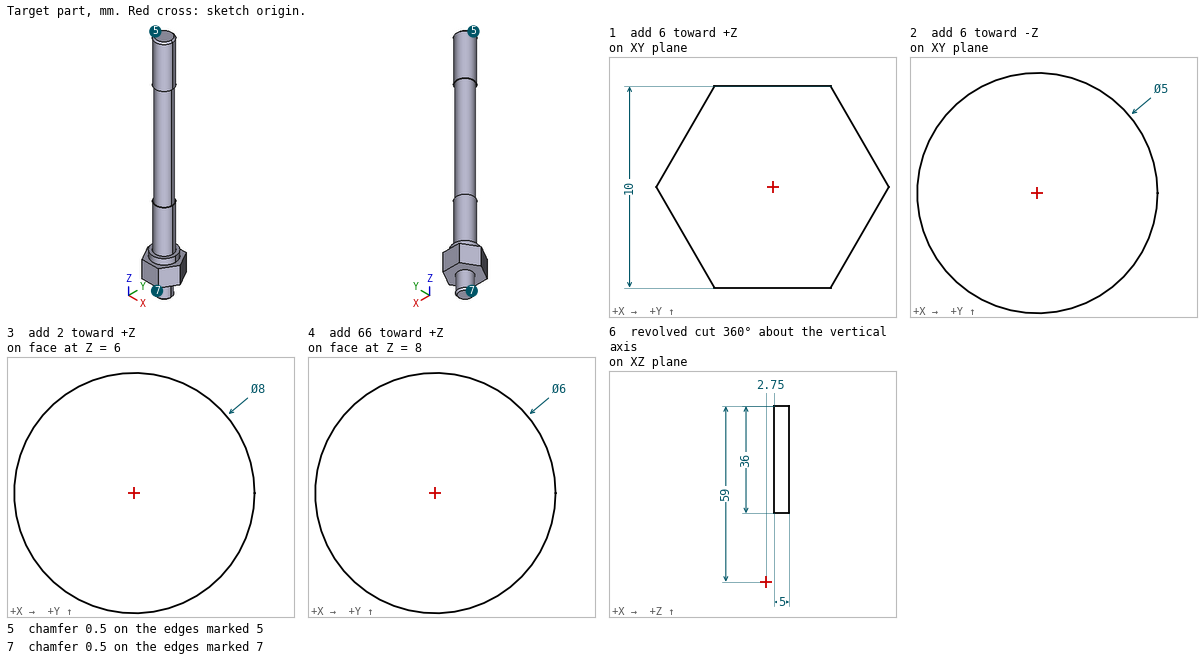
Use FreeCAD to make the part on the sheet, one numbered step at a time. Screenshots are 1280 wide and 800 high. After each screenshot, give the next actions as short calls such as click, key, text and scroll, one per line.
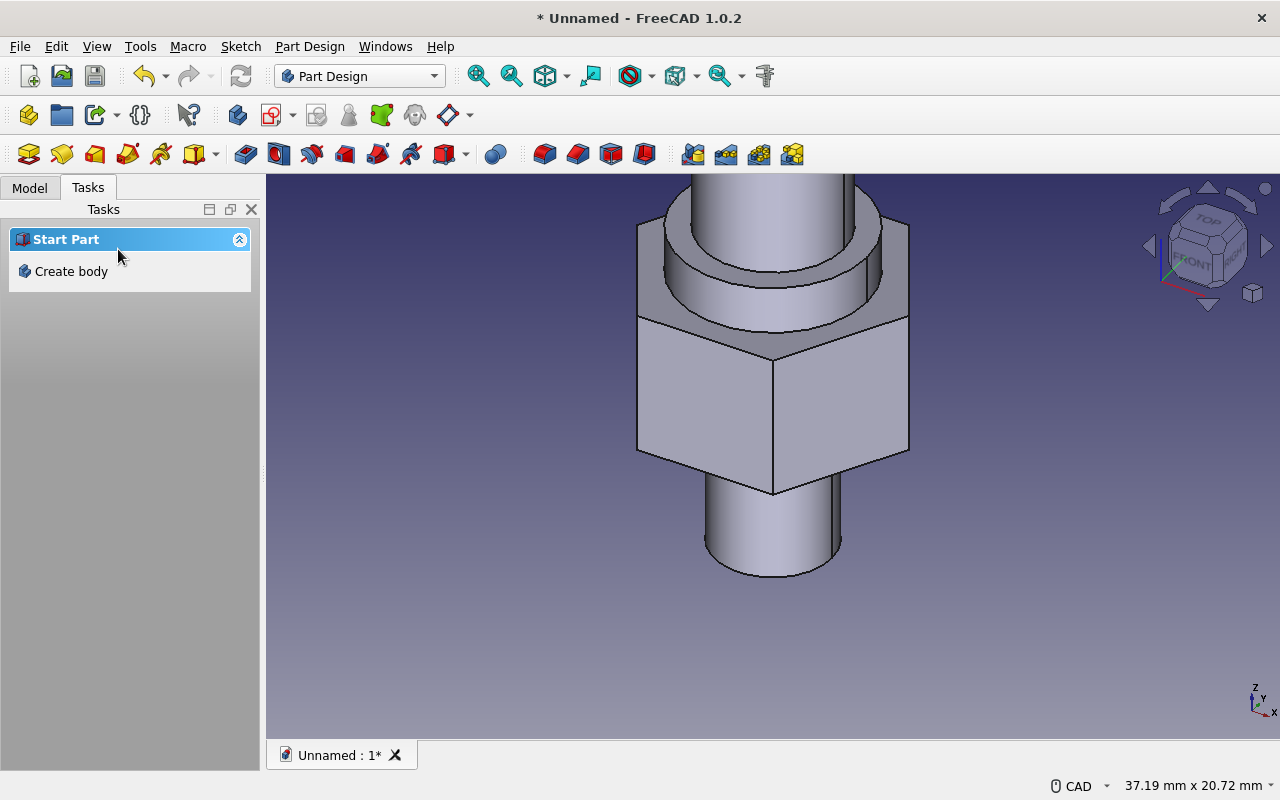
click(479, 76)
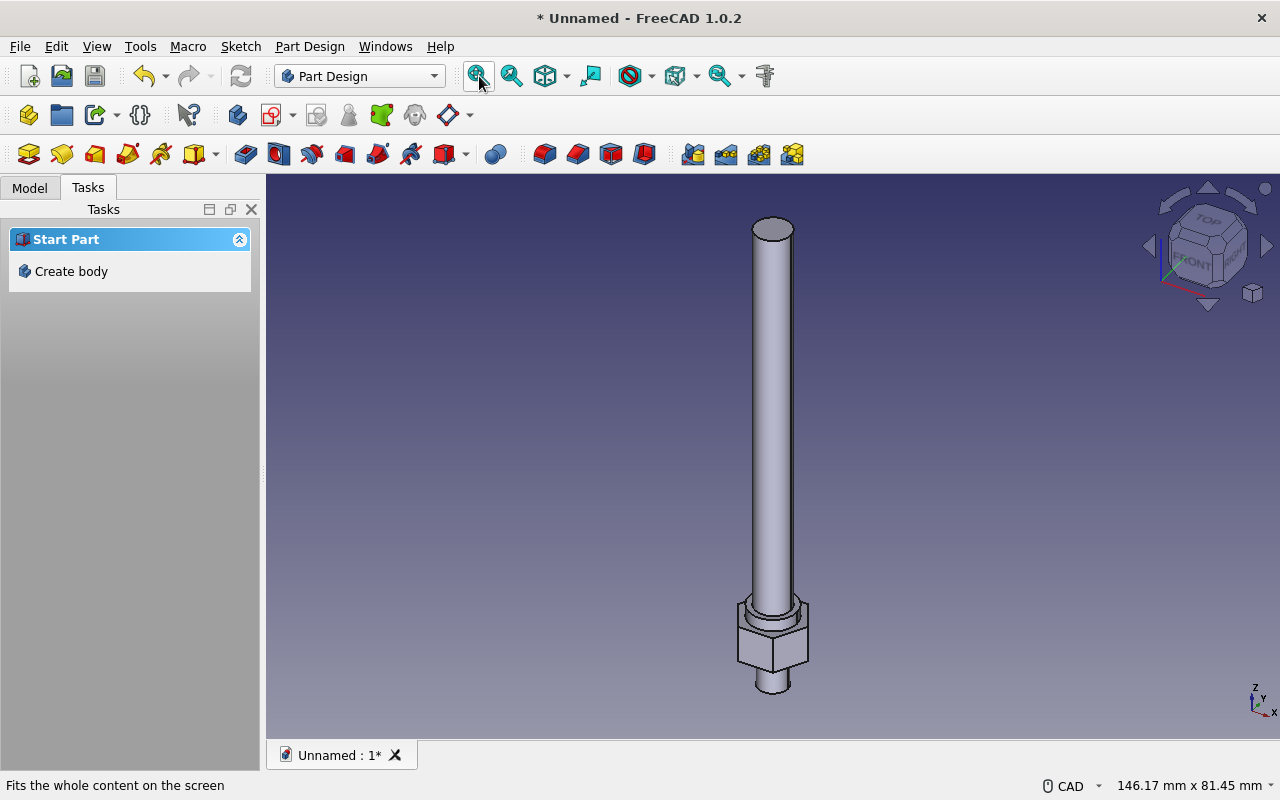
click(765, 217)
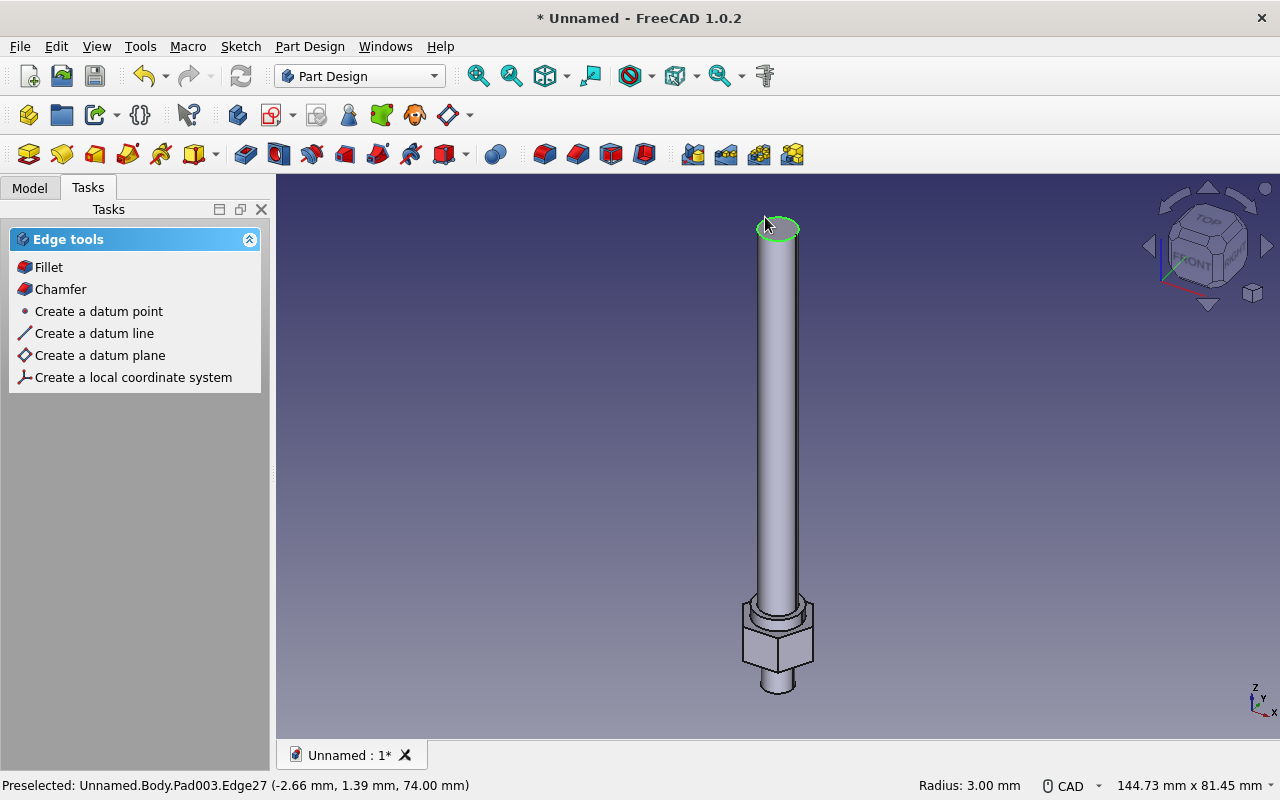
click(578, 154)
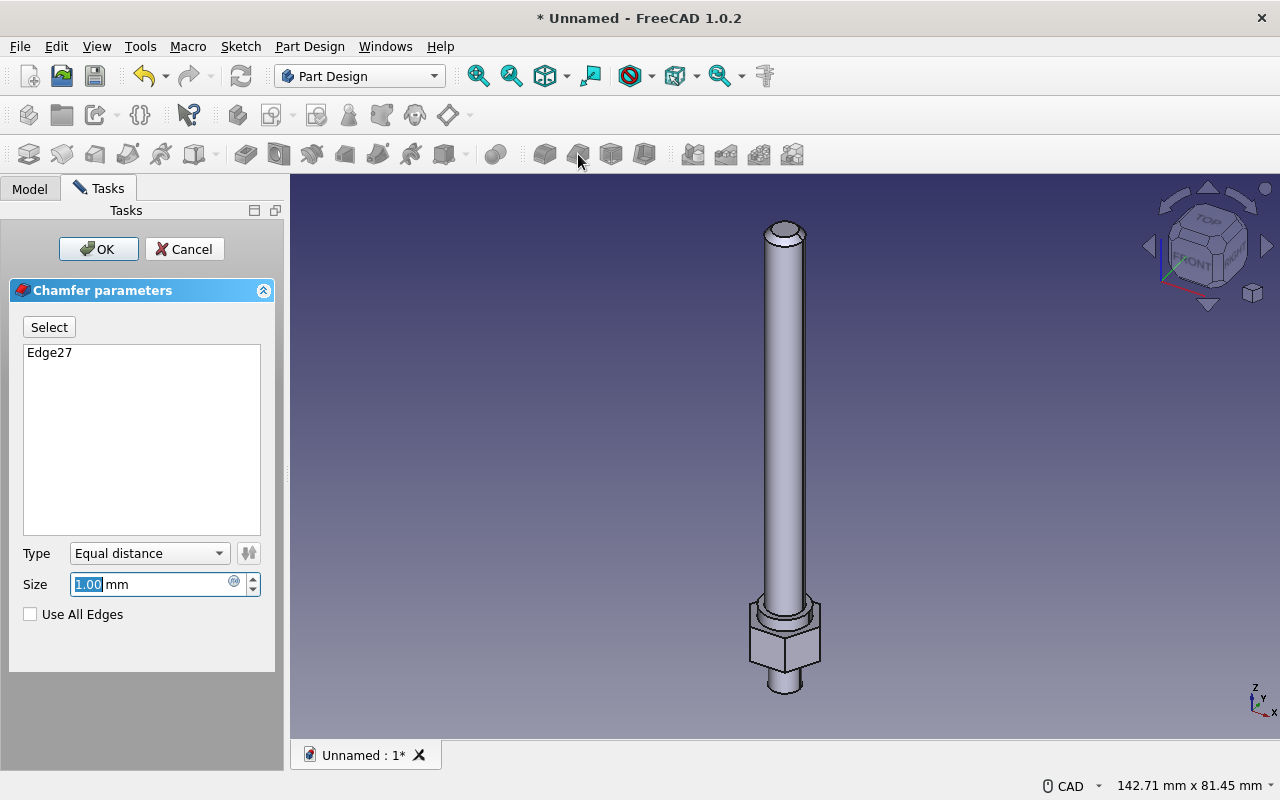
text(0.5)
key(Tab)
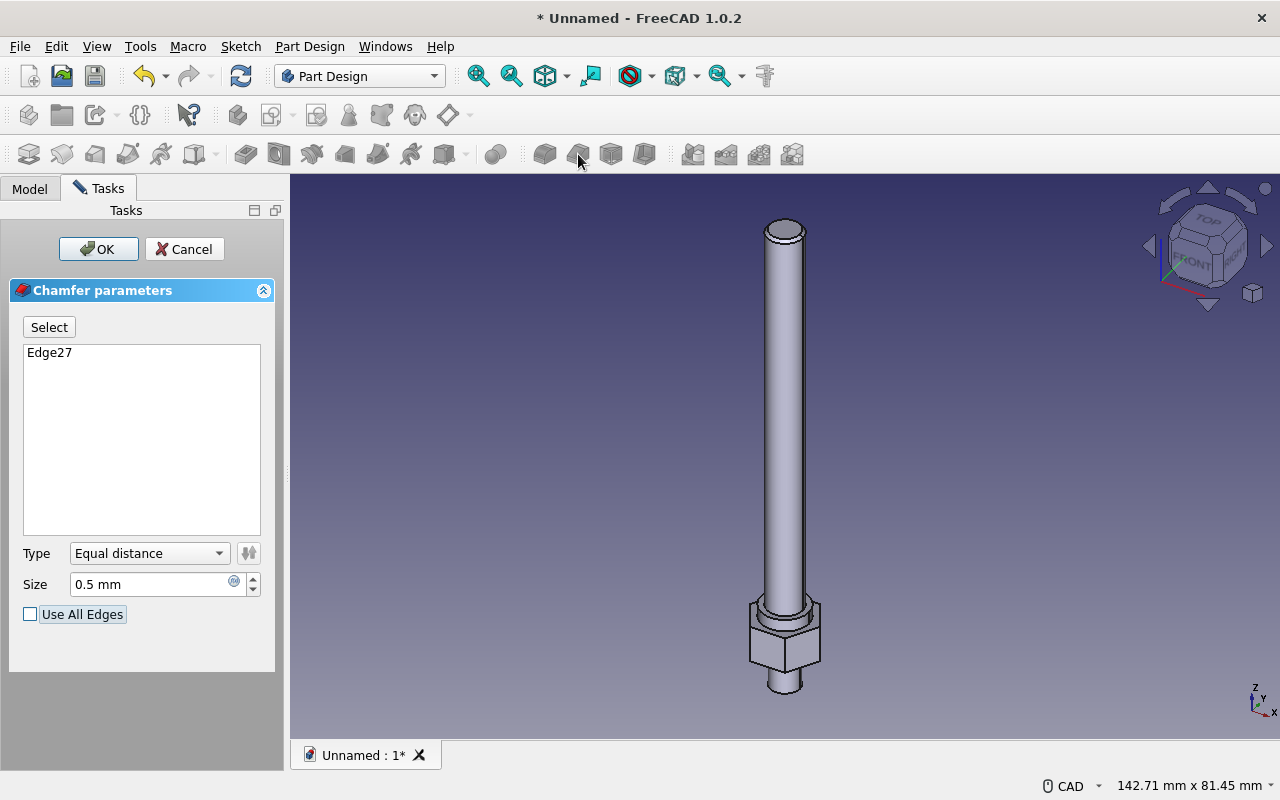
click(99, 249)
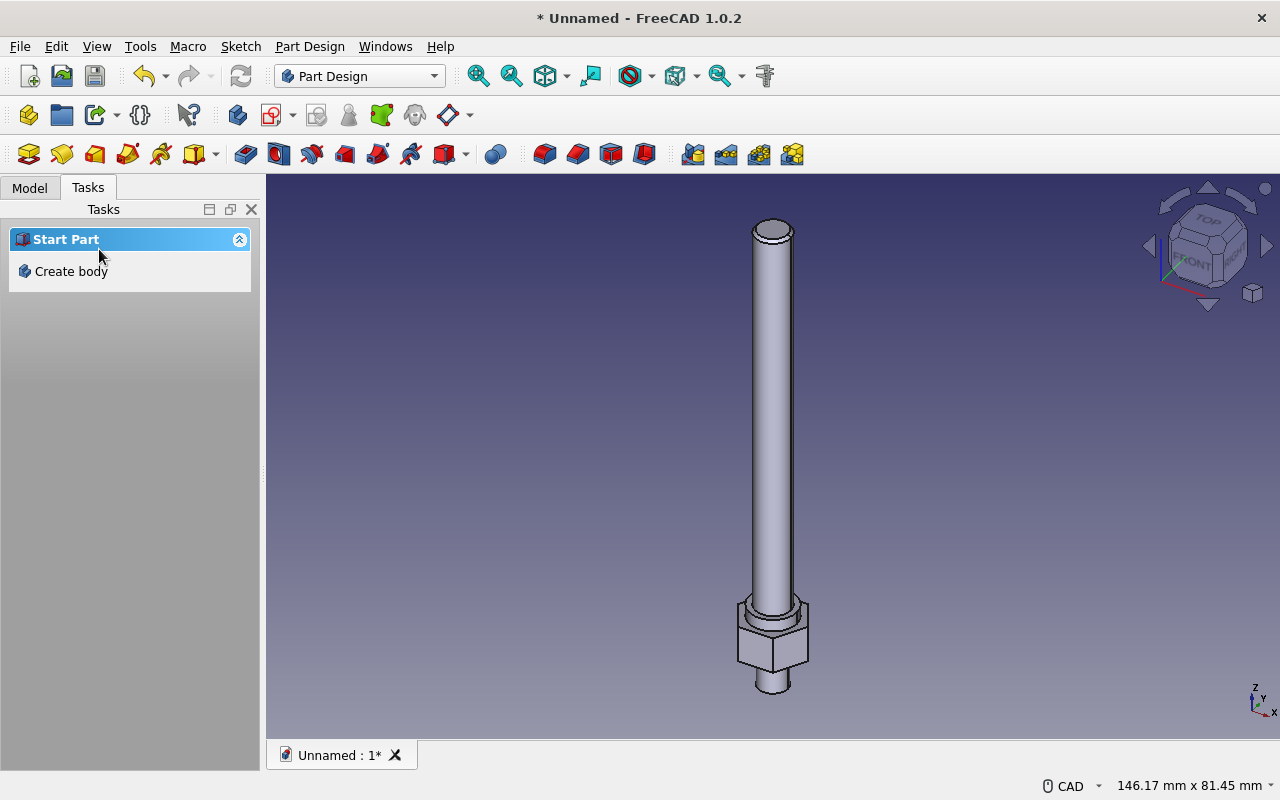
click(270, 116)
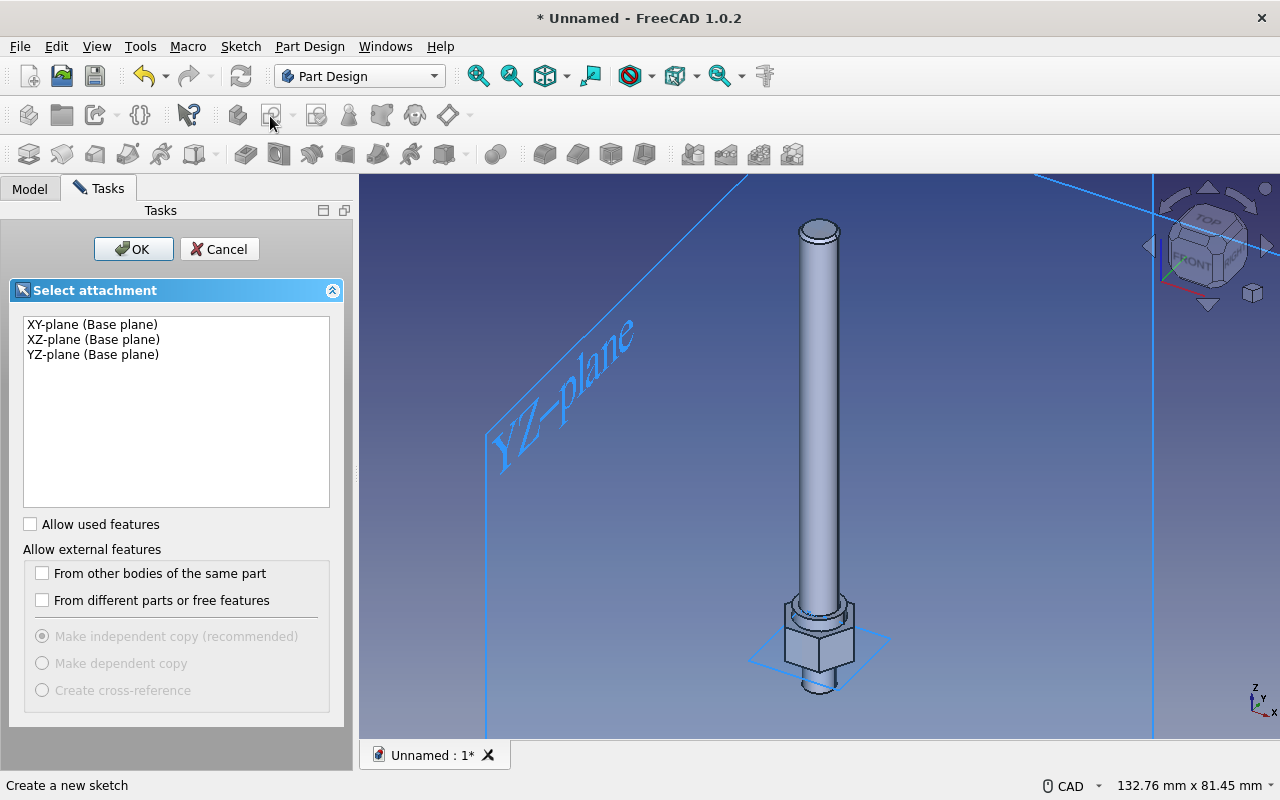
click(84, 340)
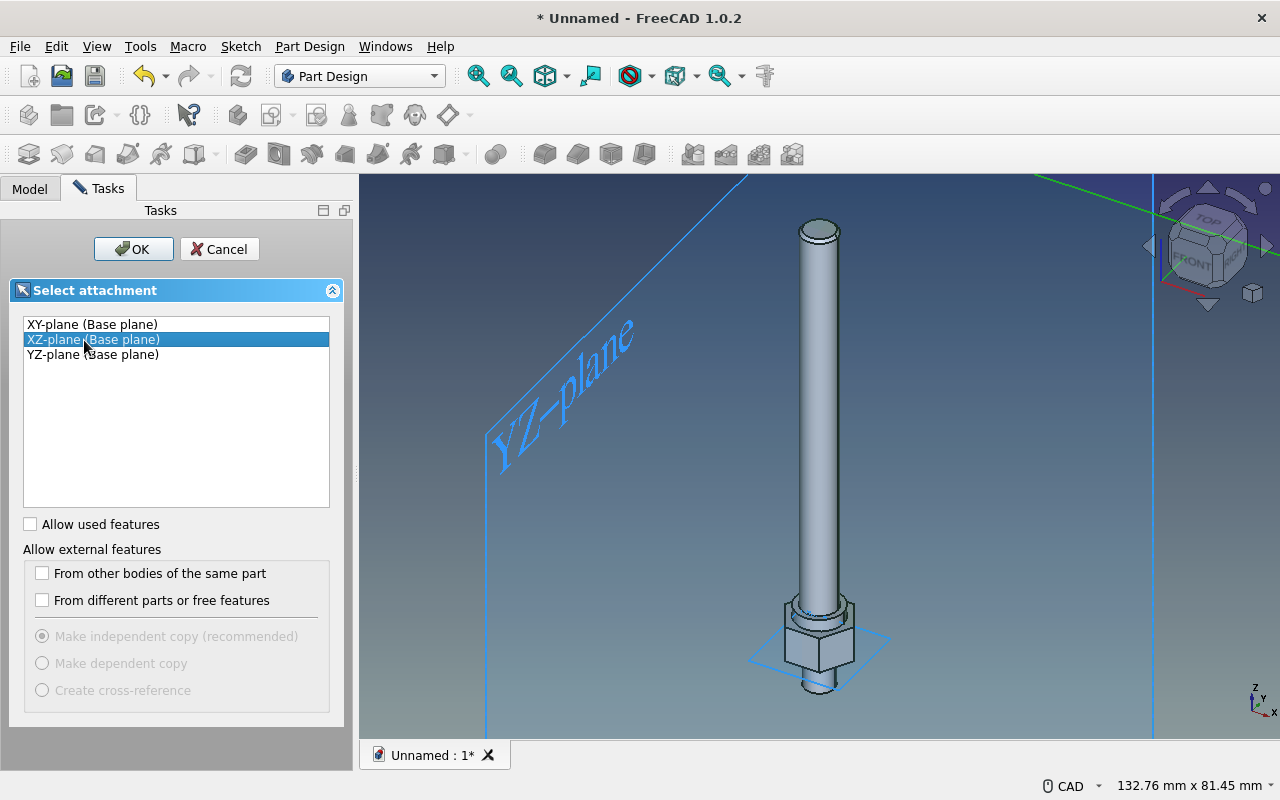
click(134, 249)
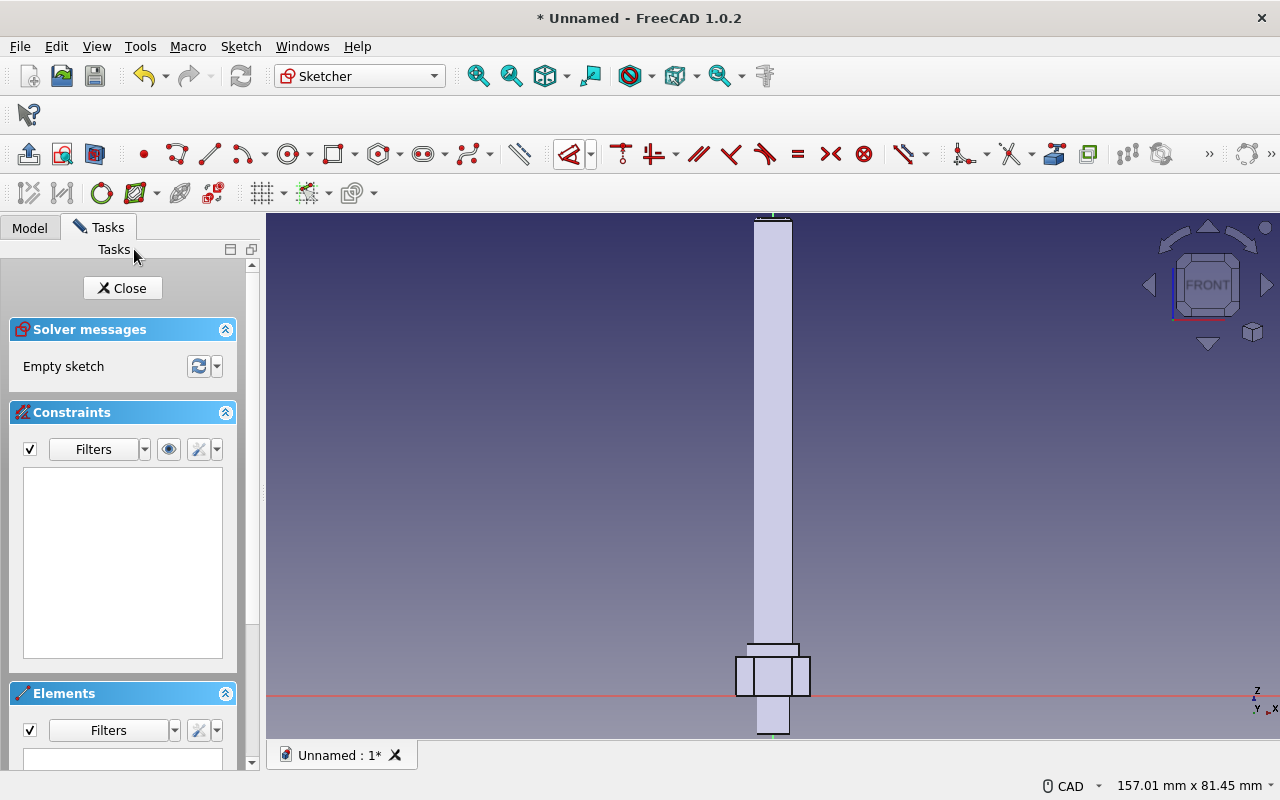
click(95, 154)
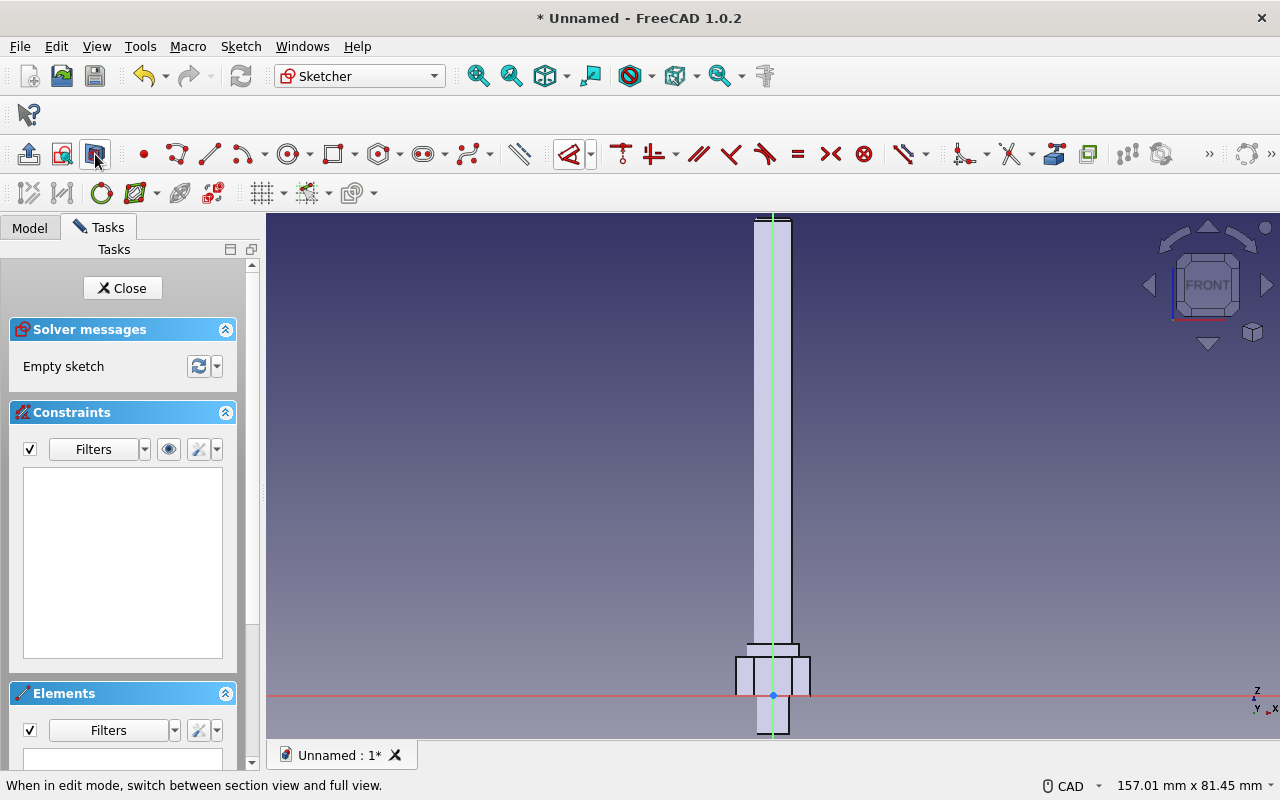
scroll(294, 345, down, 1)